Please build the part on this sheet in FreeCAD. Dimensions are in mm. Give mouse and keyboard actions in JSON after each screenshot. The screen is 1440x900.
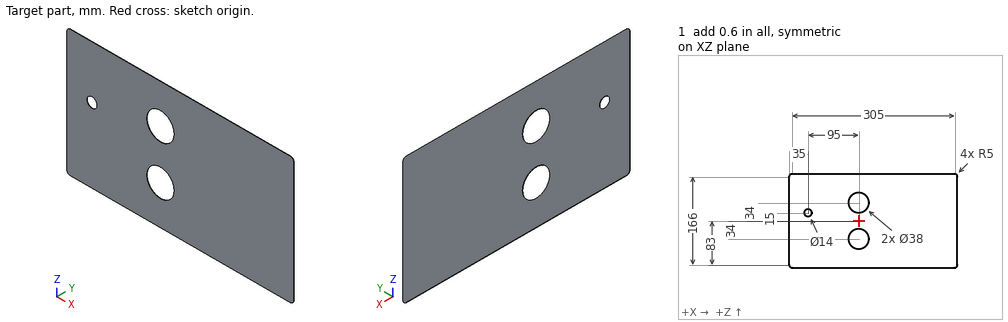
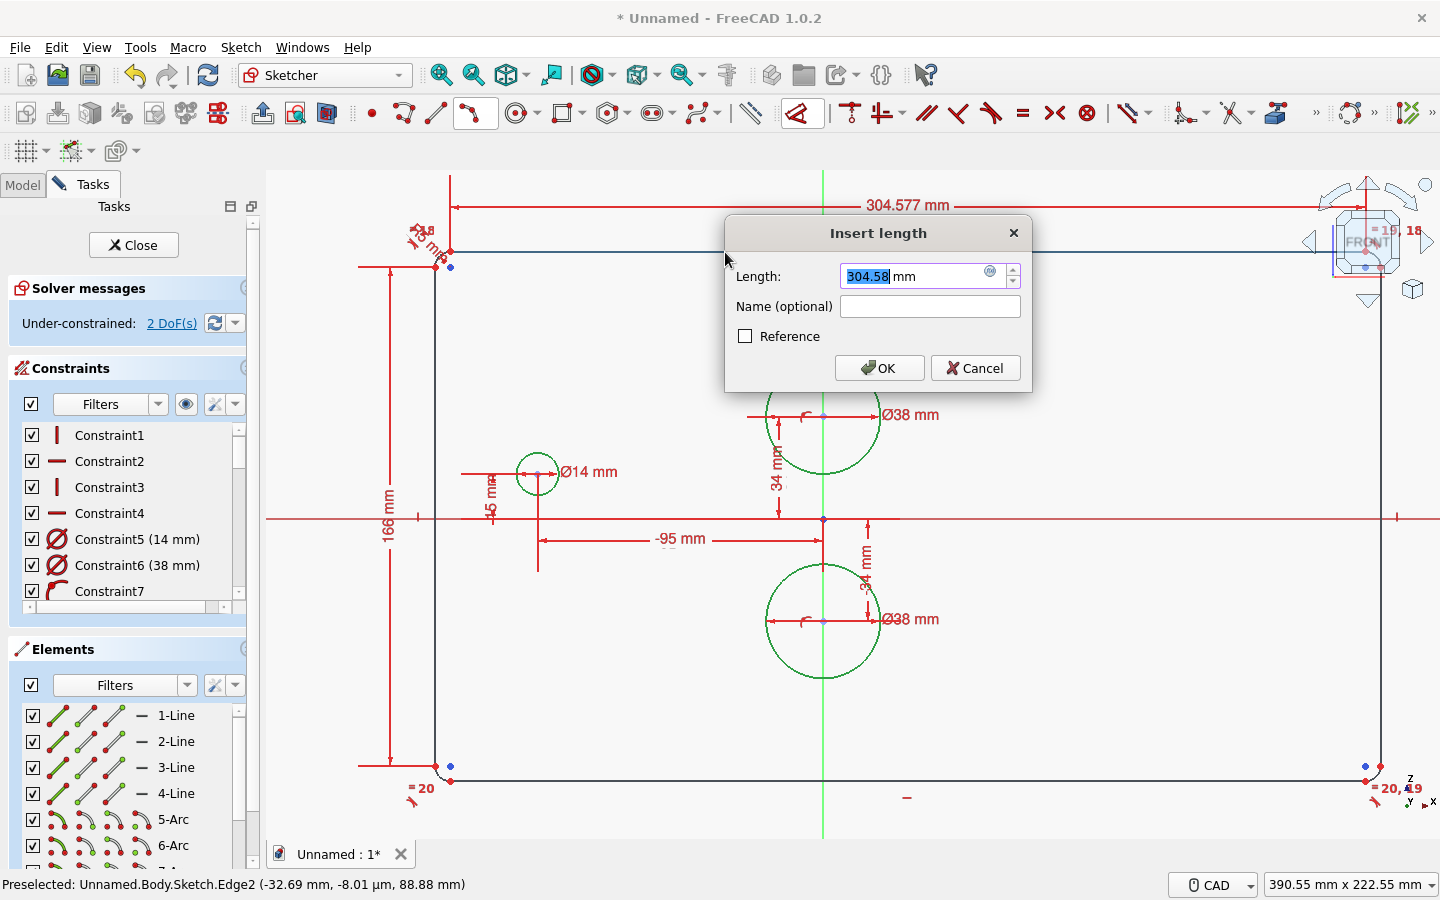
{"action": "type", "text": "305"}
{"action": "key", "text": "Return"}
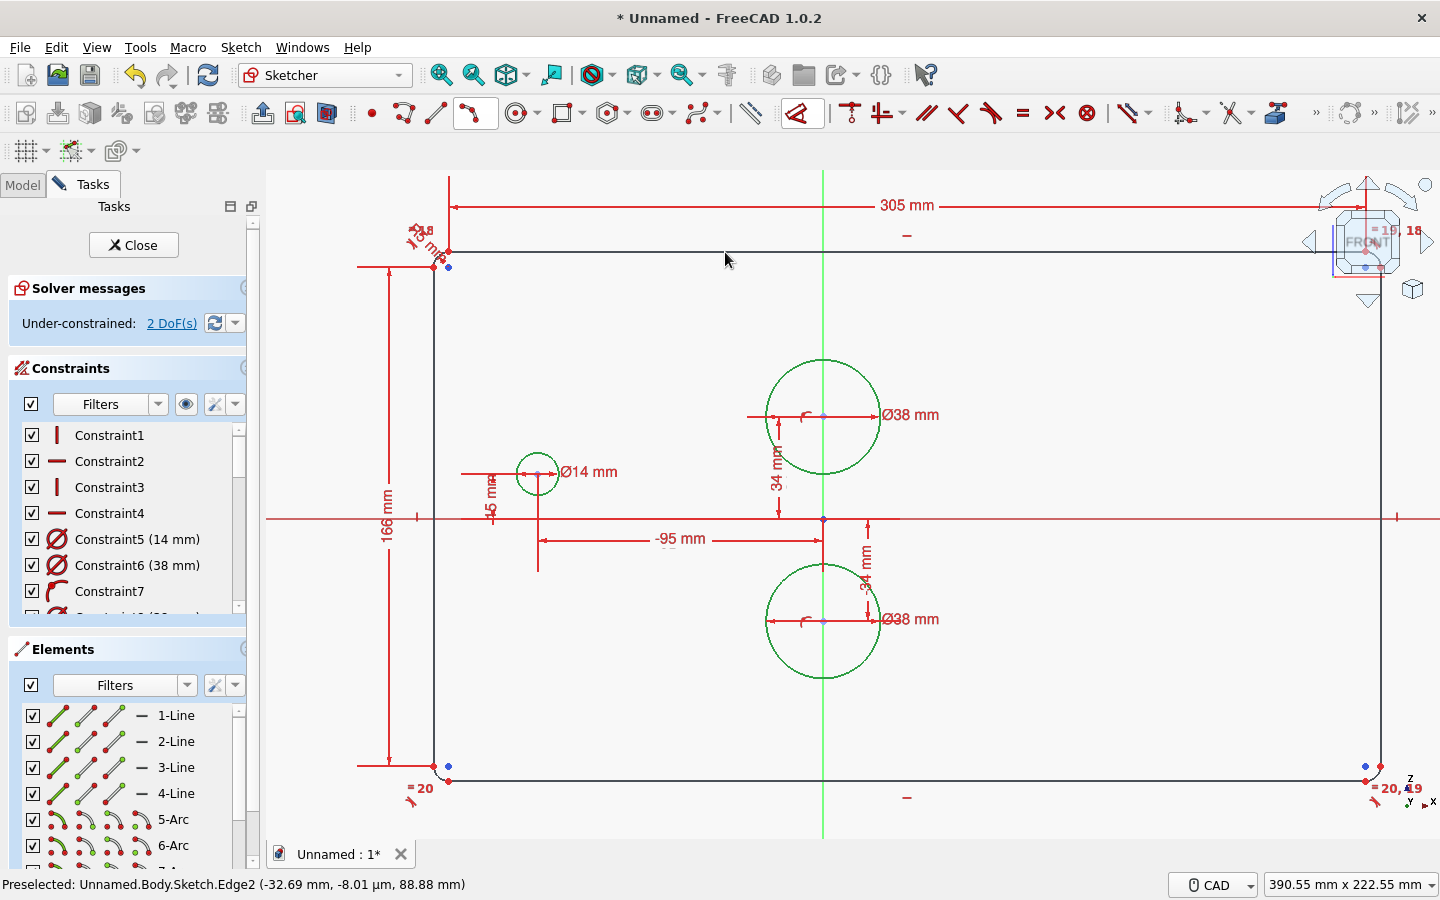
{"action": "left_click", "coordinate": [434, 766]}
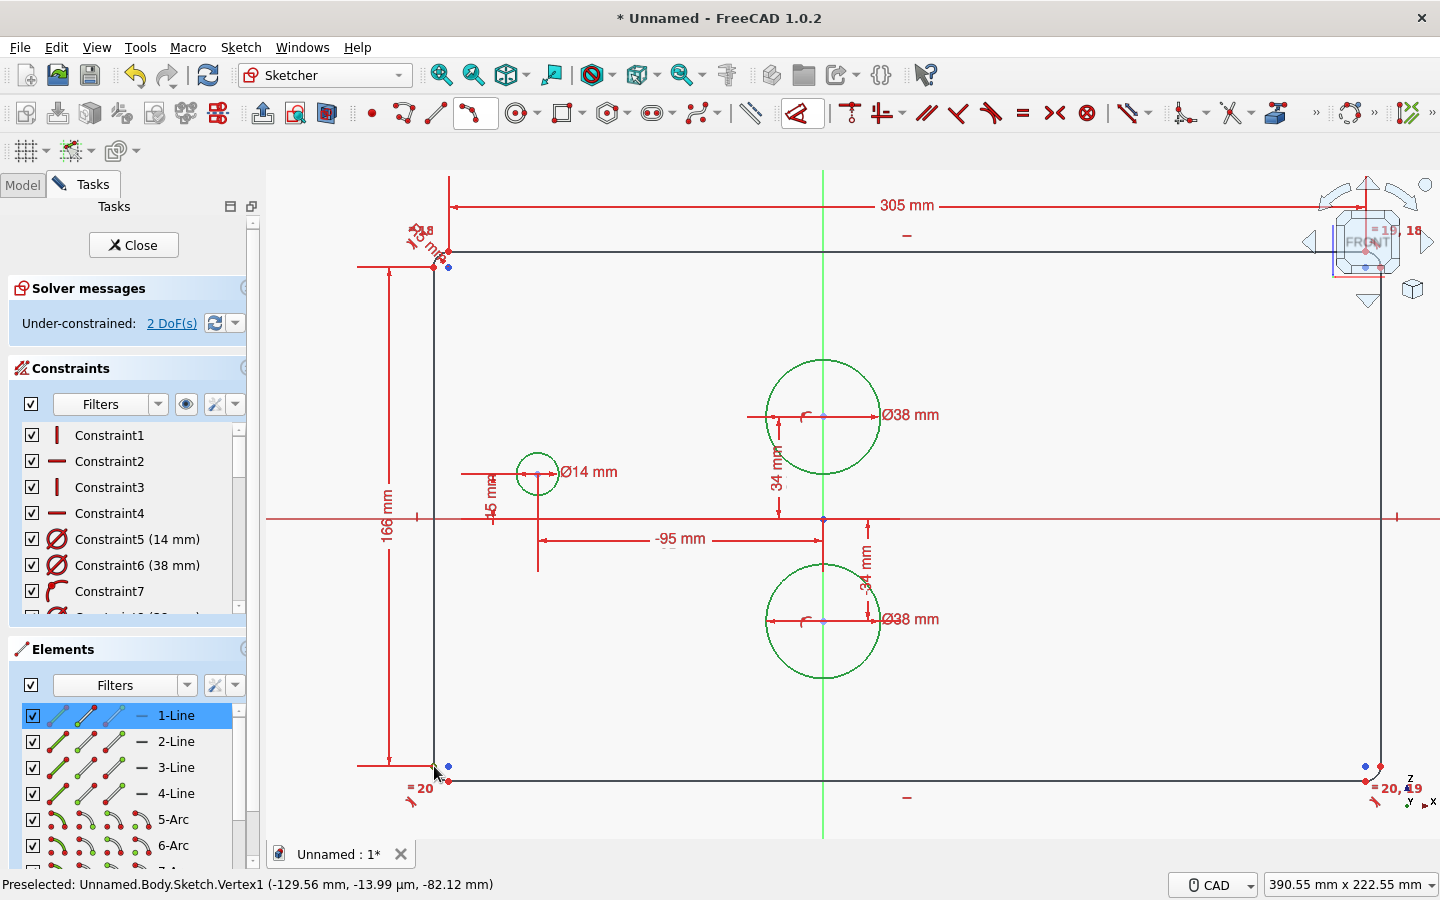
{"action": "left_click", "coordinate": [818, 114]}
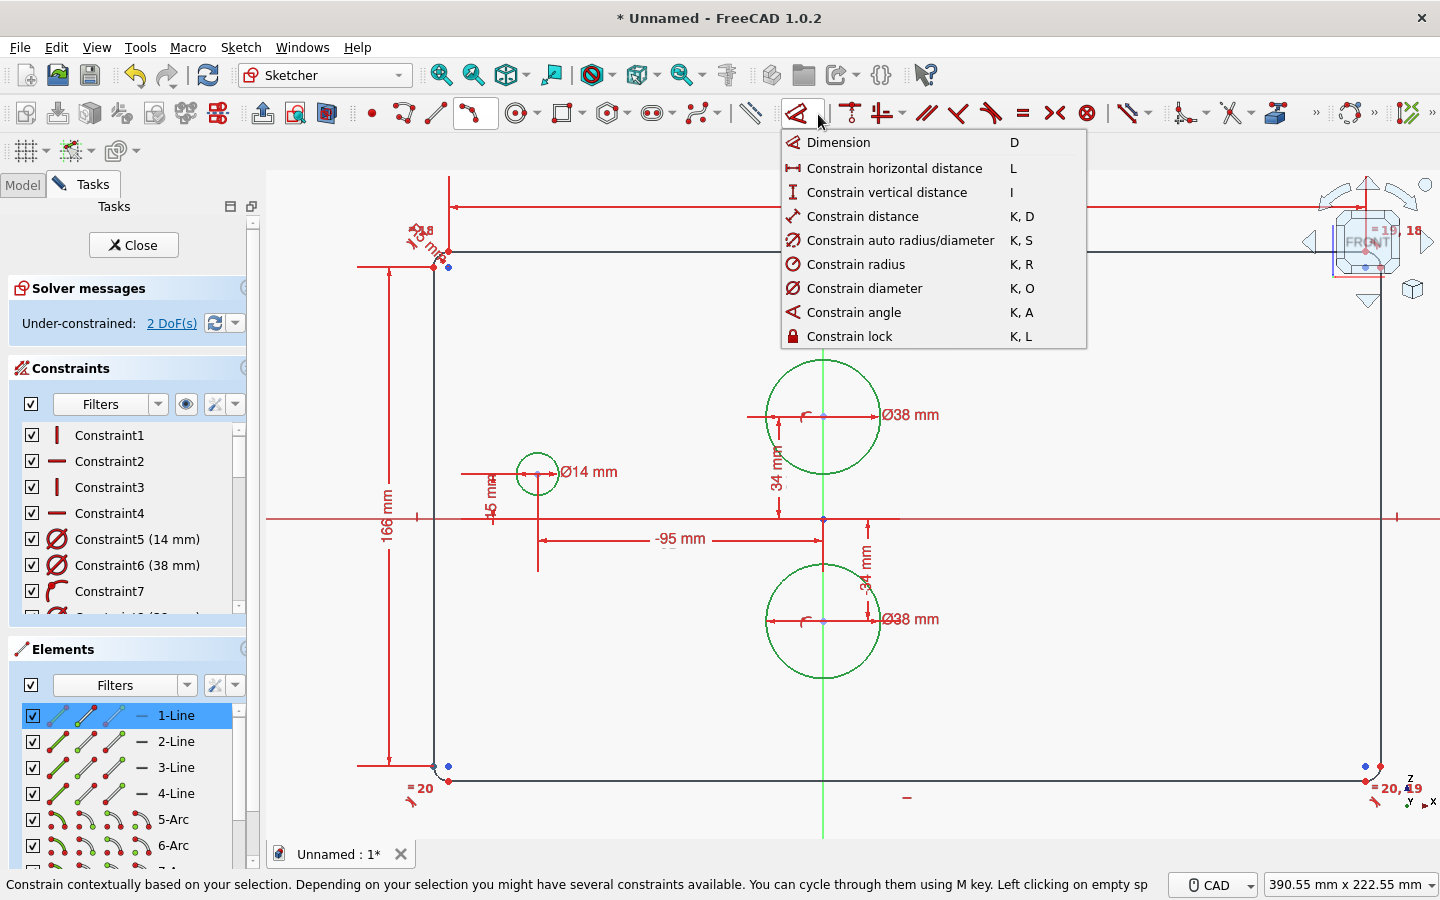
{"action": "left_click", "coordinate": [934, 192]}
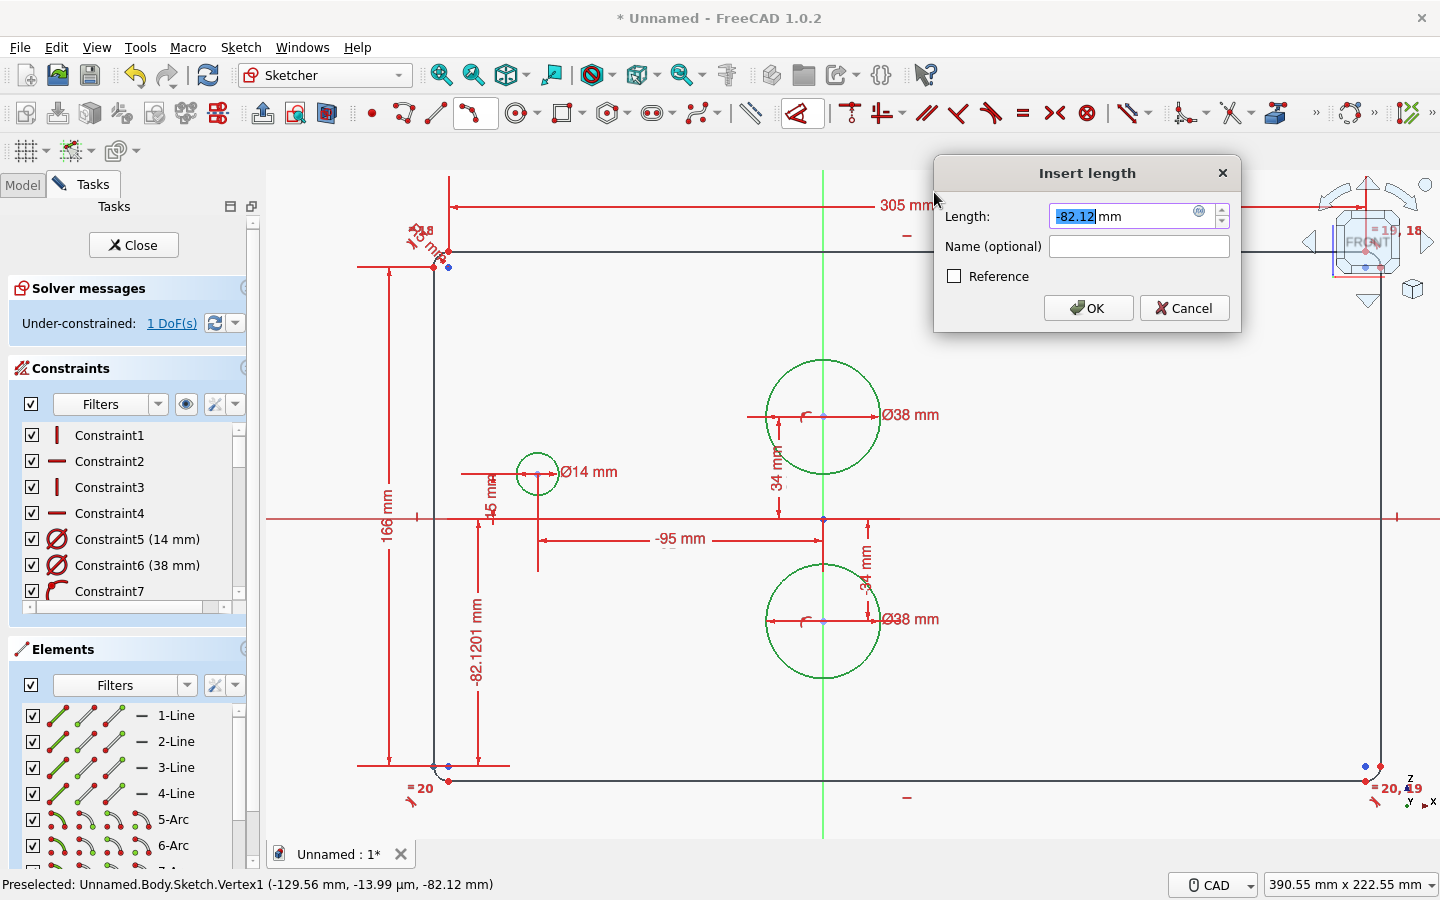
{"action": "type", "text": "-83"}
{"action": "key", "text": "Return"}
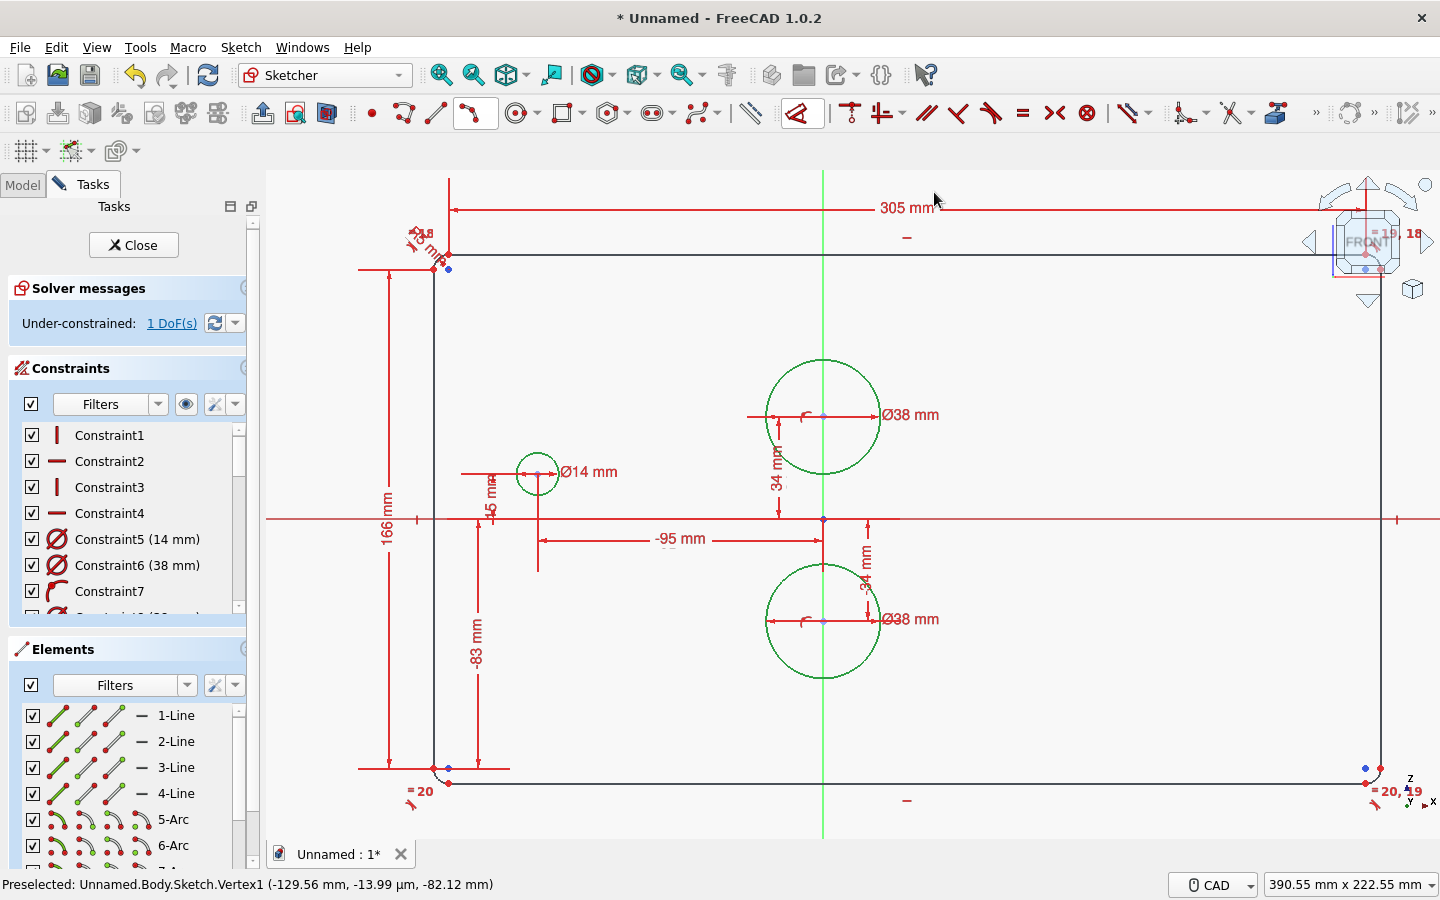
{"action": "left_click", "coordinate": [434, 270]}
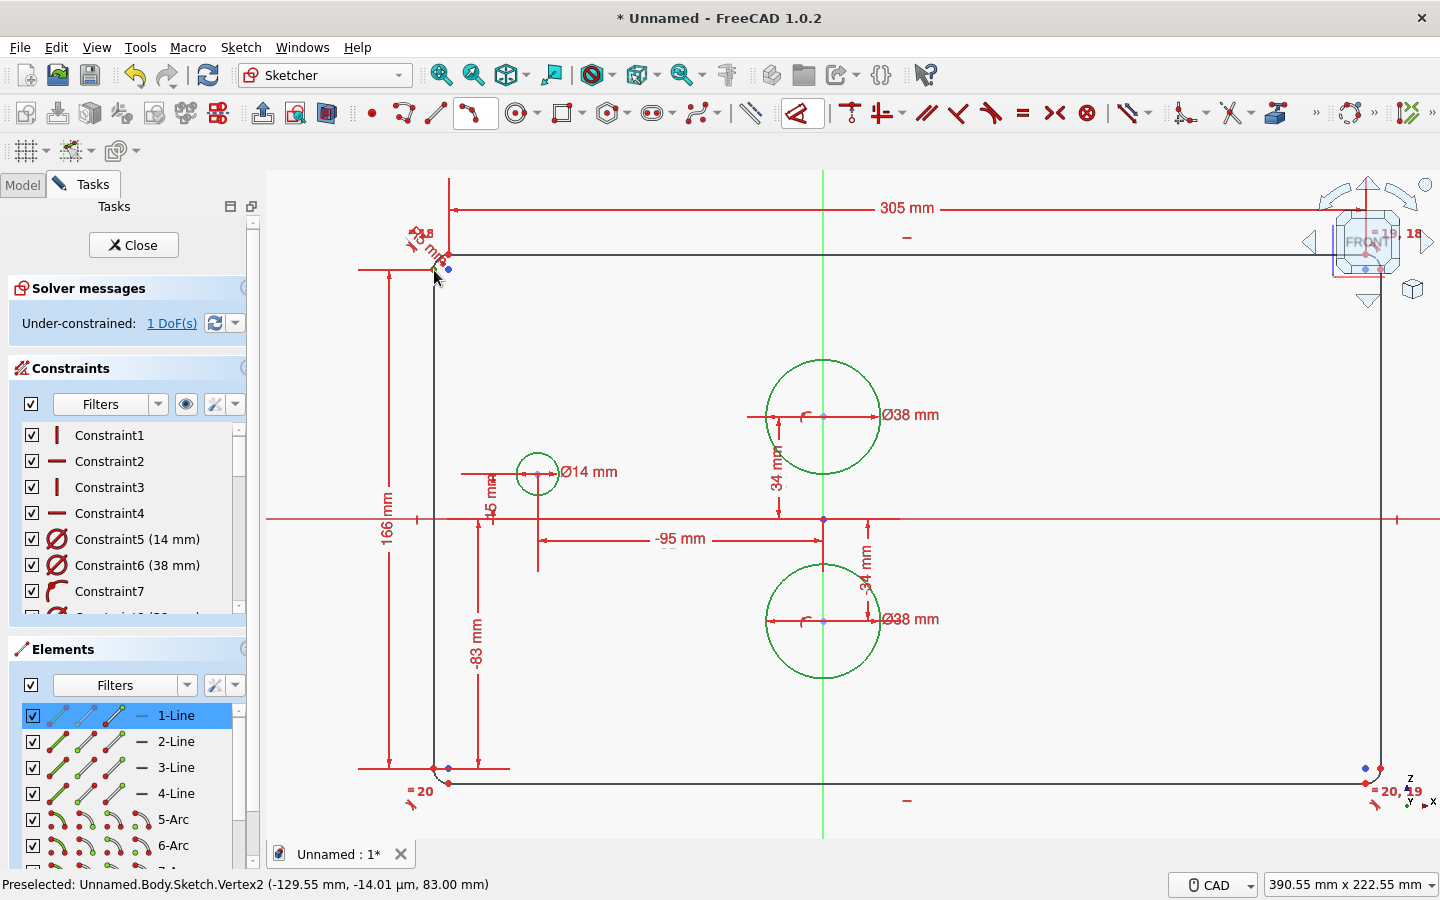
{"action": "left_click", "coordinate": [538, 474]}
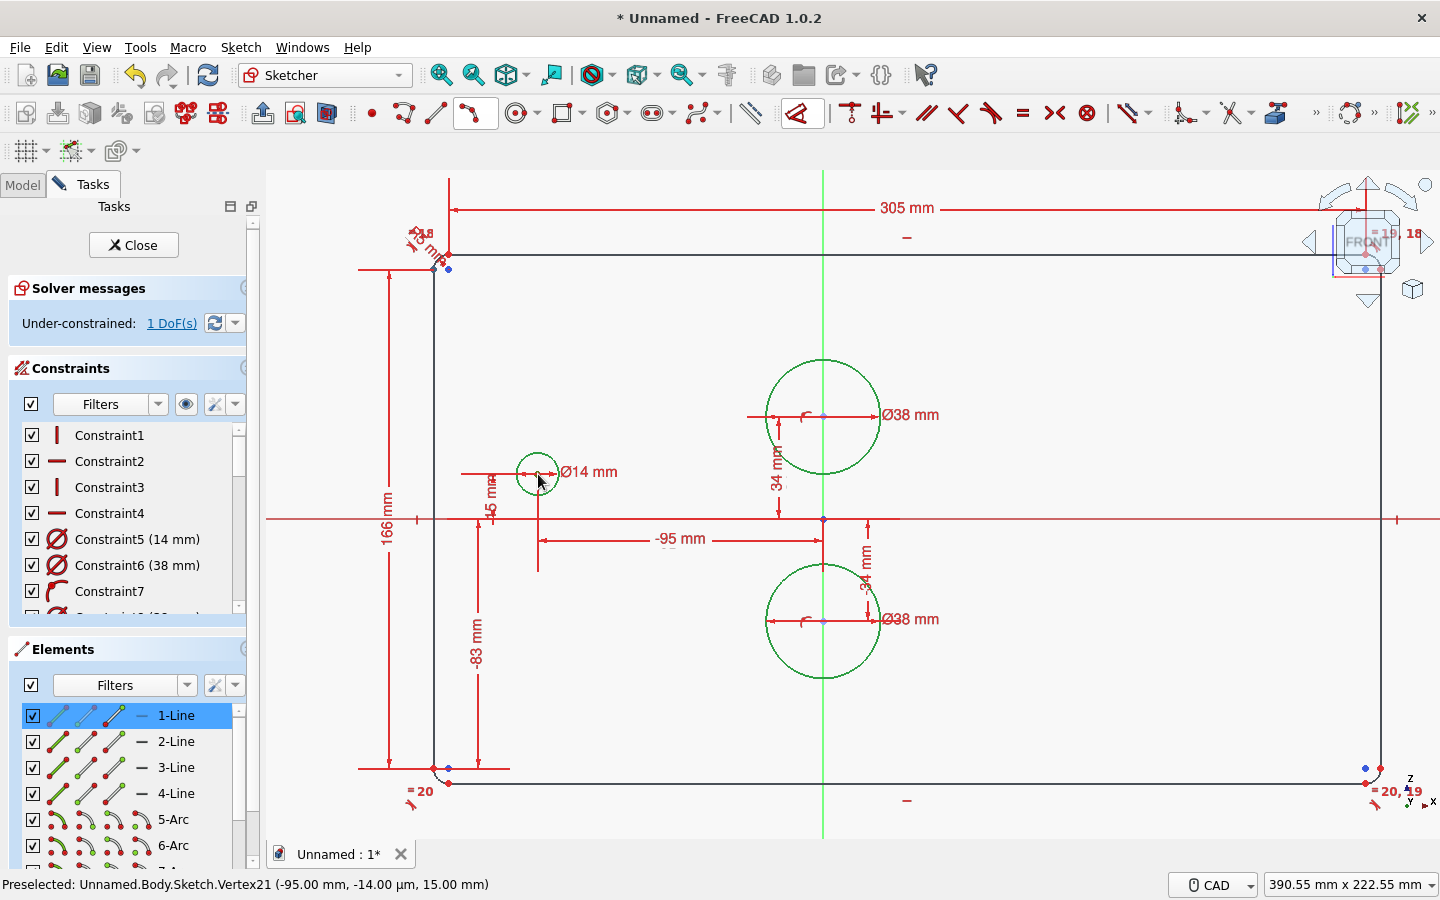
{"action": "key", "text": "l"}